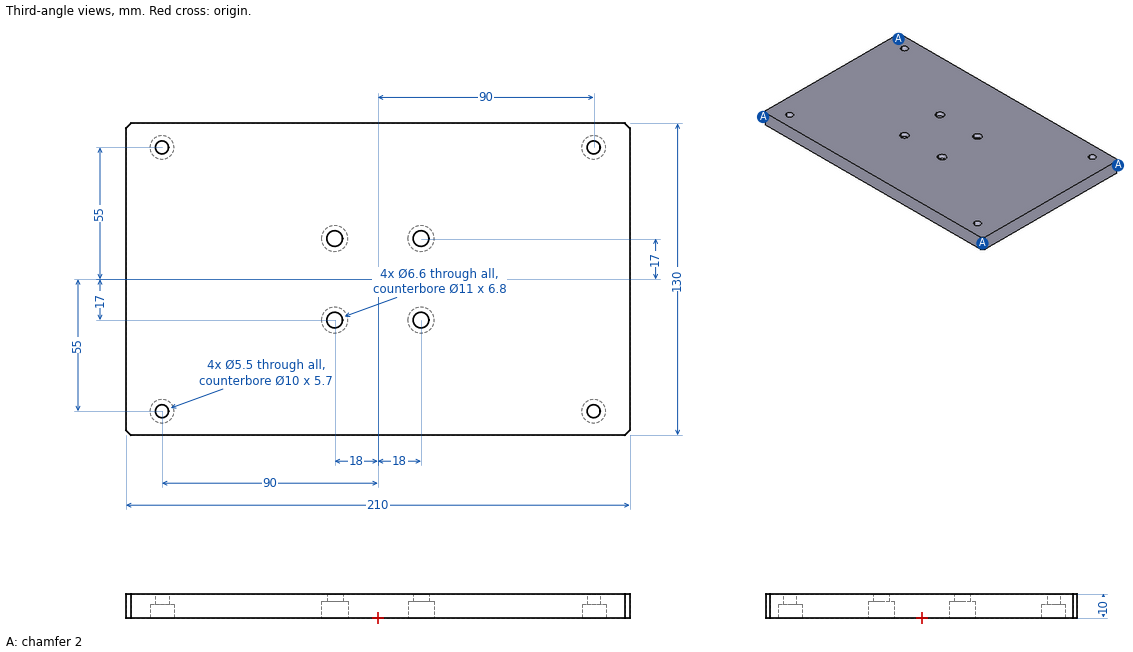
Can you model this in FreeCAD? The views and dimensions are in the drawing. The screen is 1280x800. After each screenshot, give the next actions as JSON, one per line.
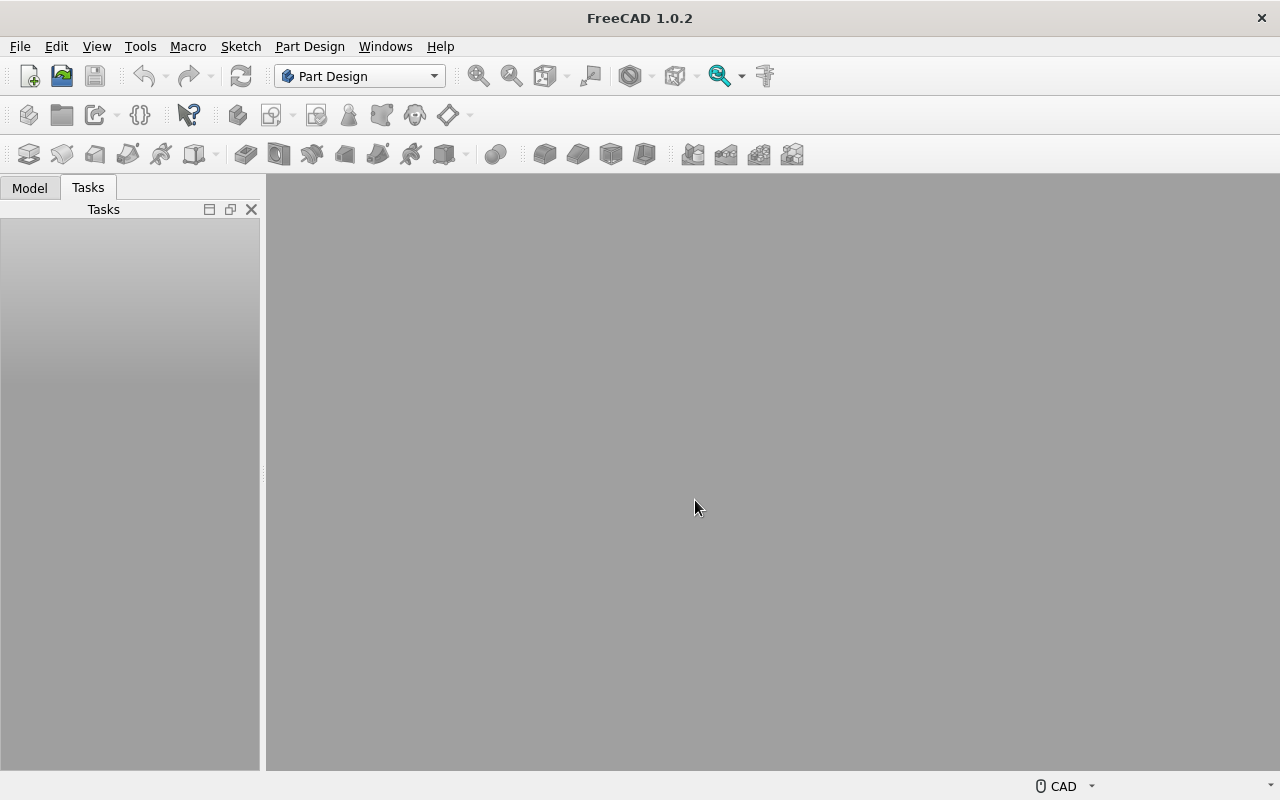
{"action": "left_click", "coordinate": [29, 76]}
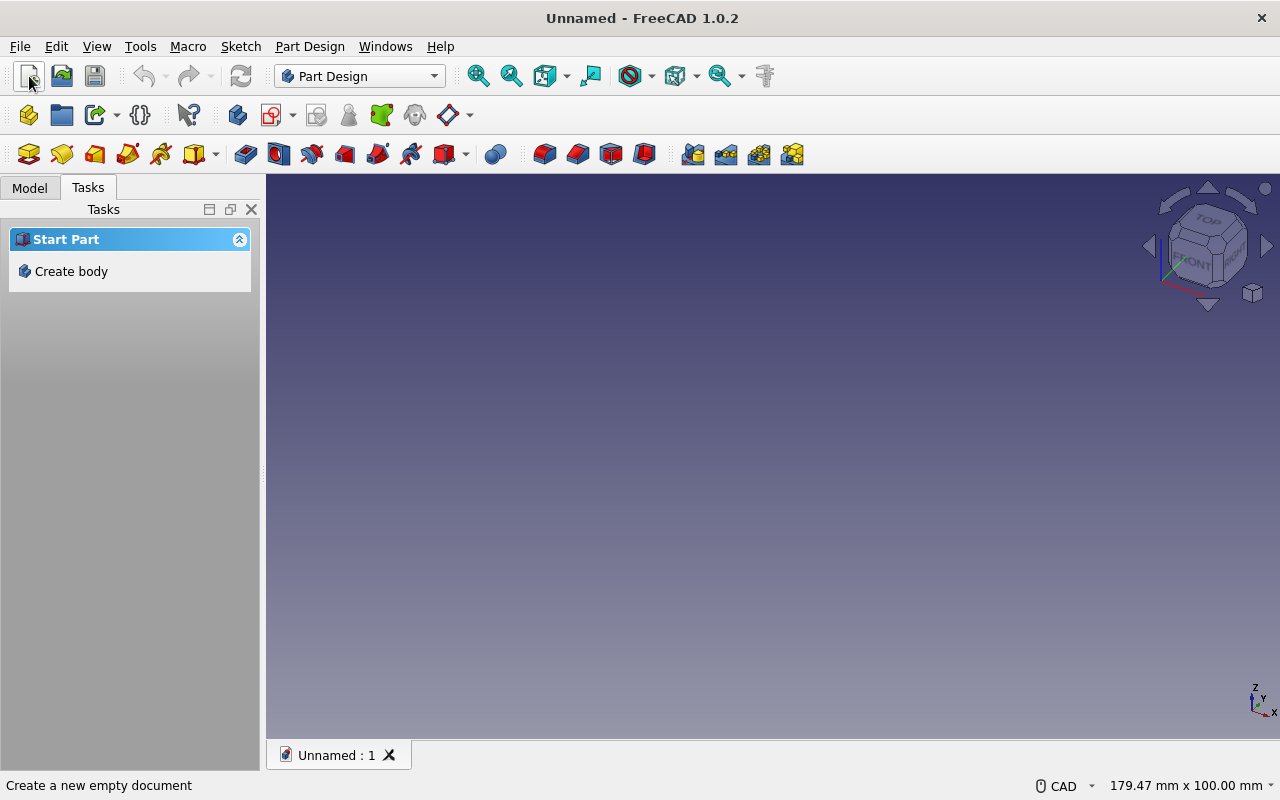
{"action": "left_click", "coordinate": [270, 116]}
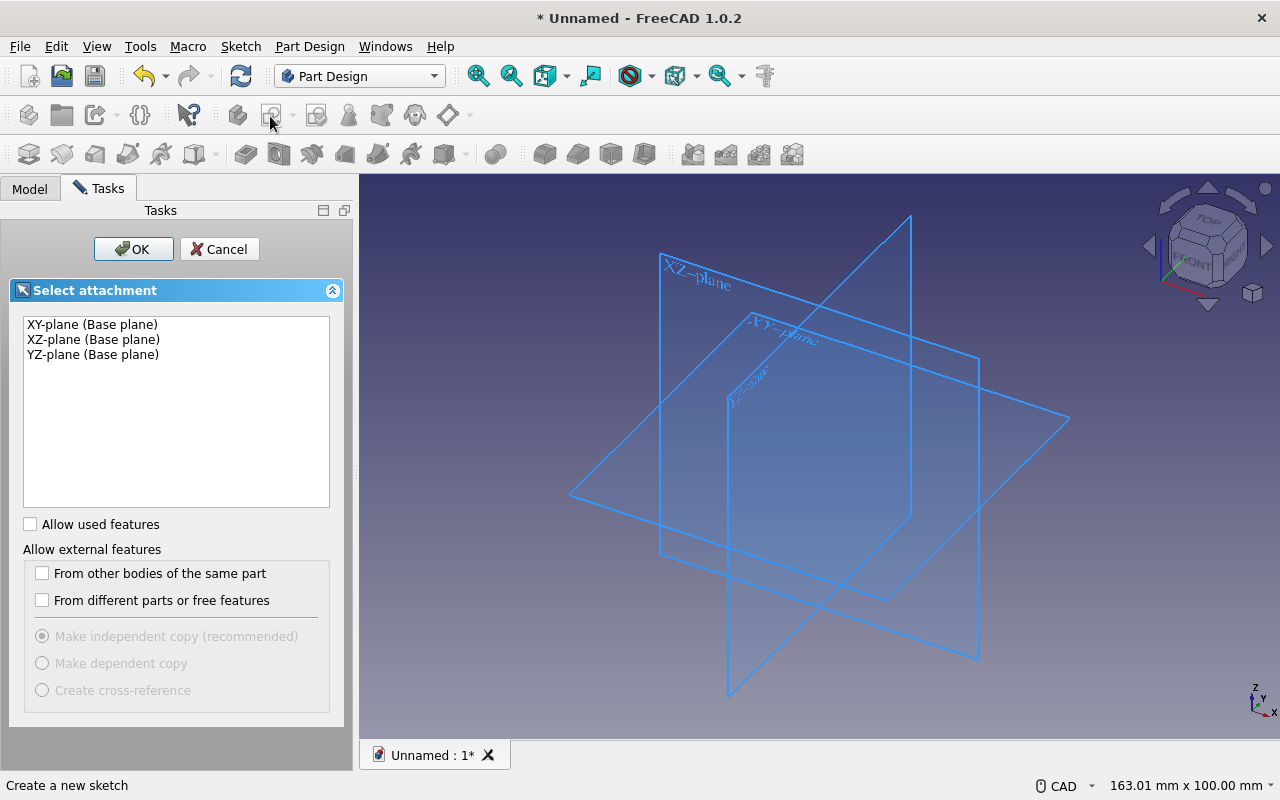
{"action": "left_click", "coordinate": [84, 324]}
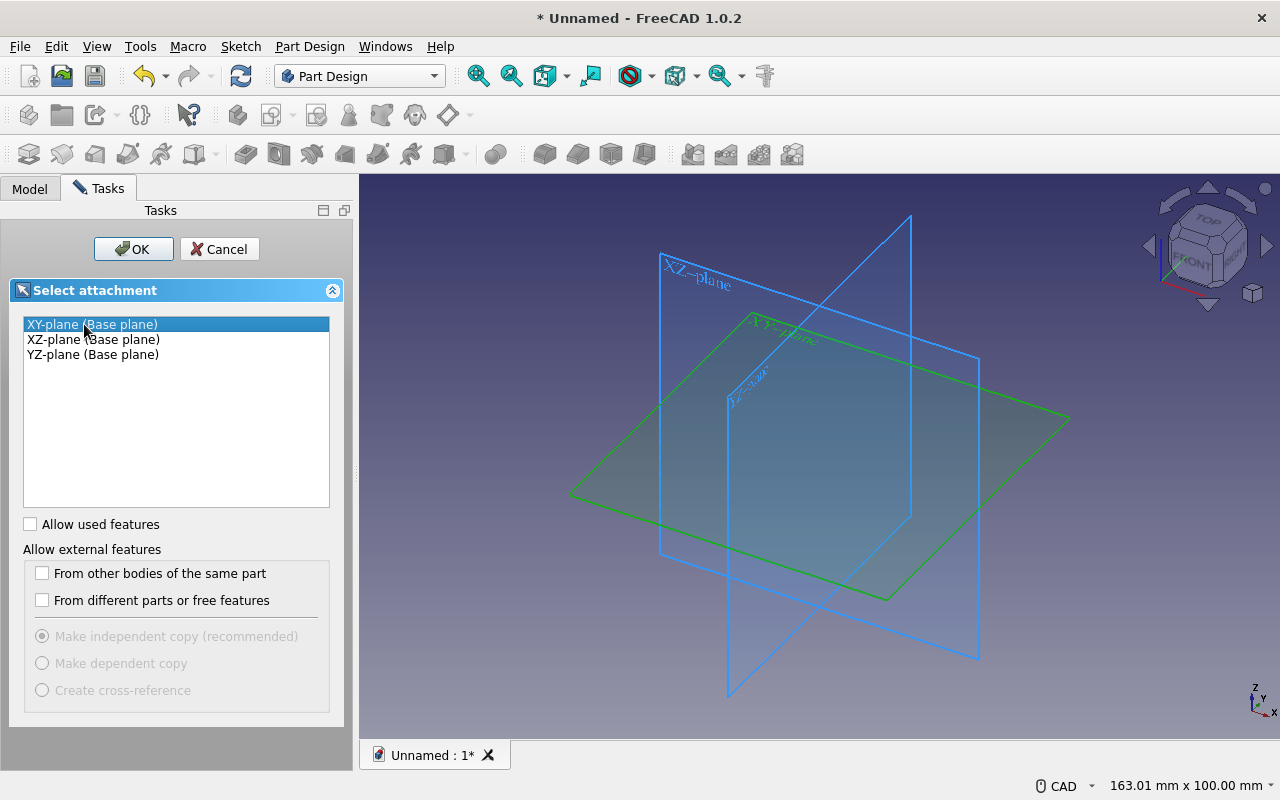
{"action": "left_click", "coordinate": [134, 249]}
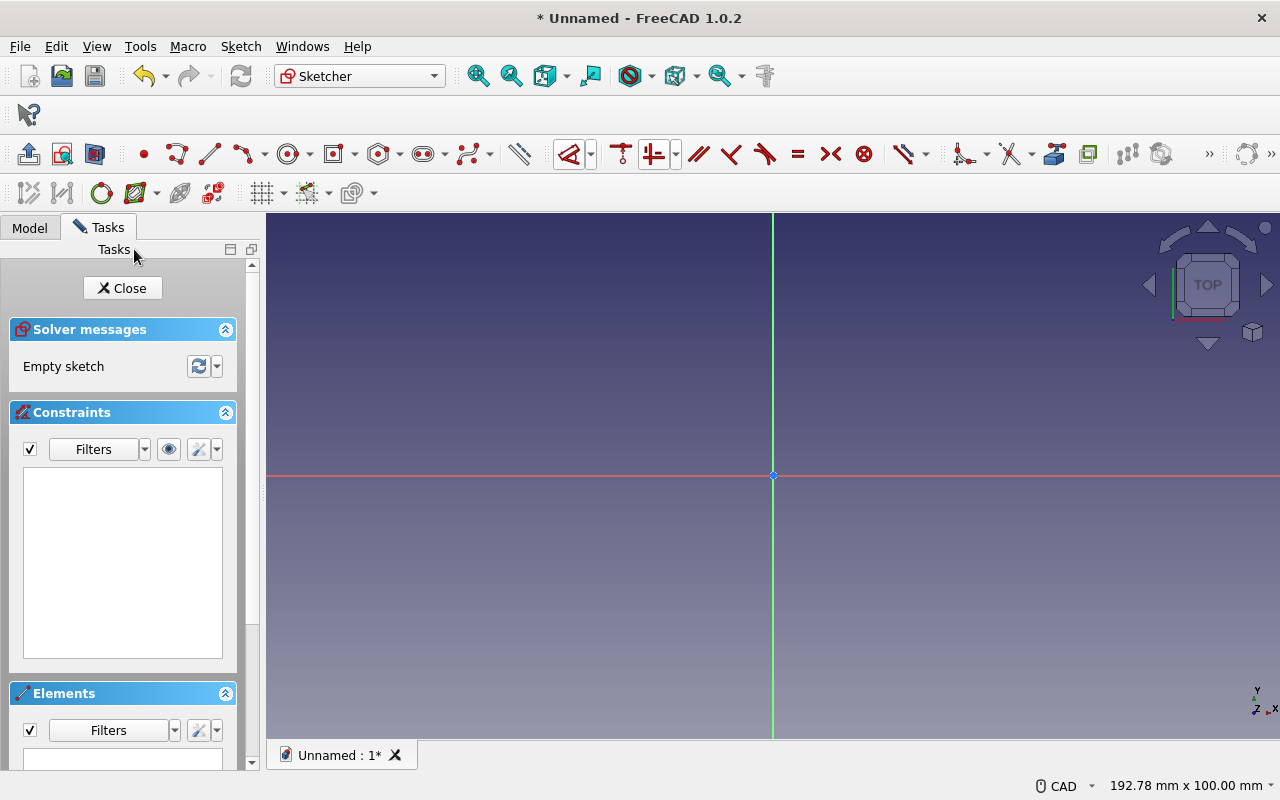
{"action": "scroll", "coordinate": [649, 476], "scroll_direction": "down", "scroll_amount": 4}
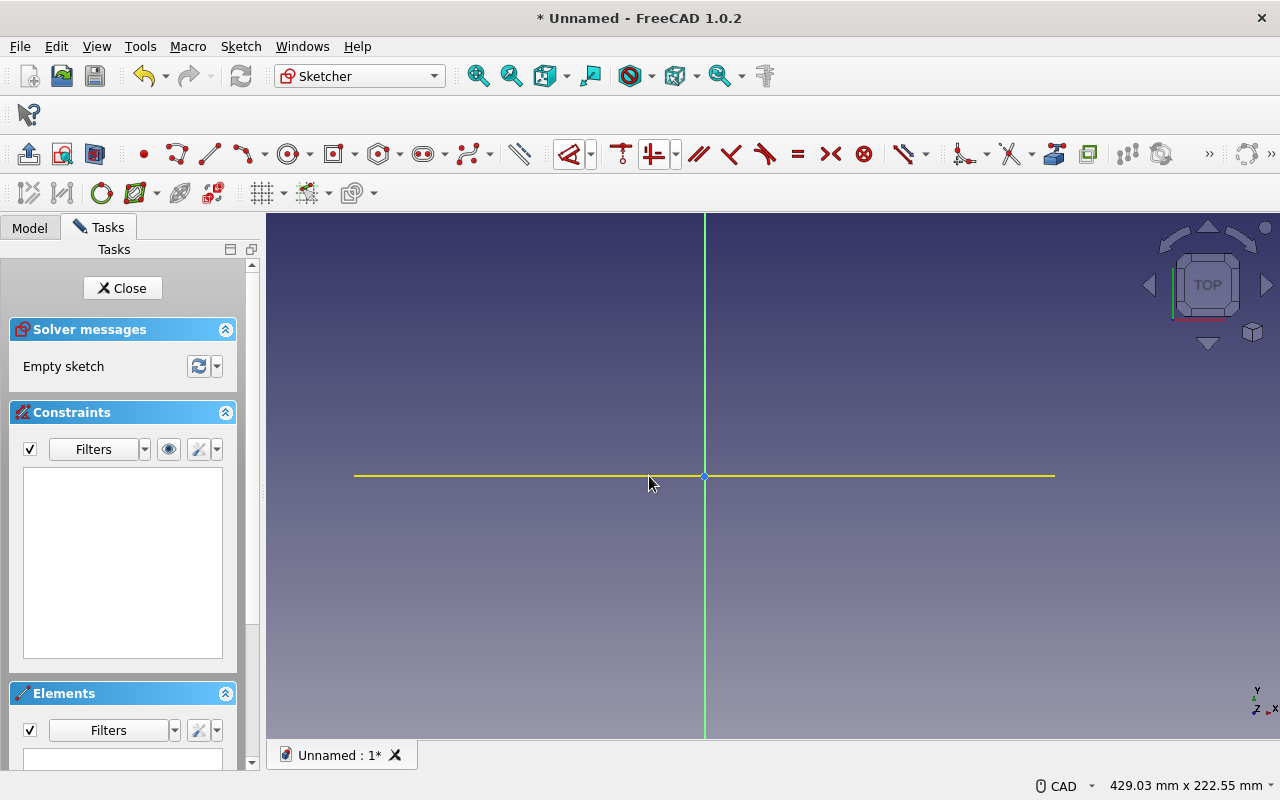
{"action": "key", "text": "g v"}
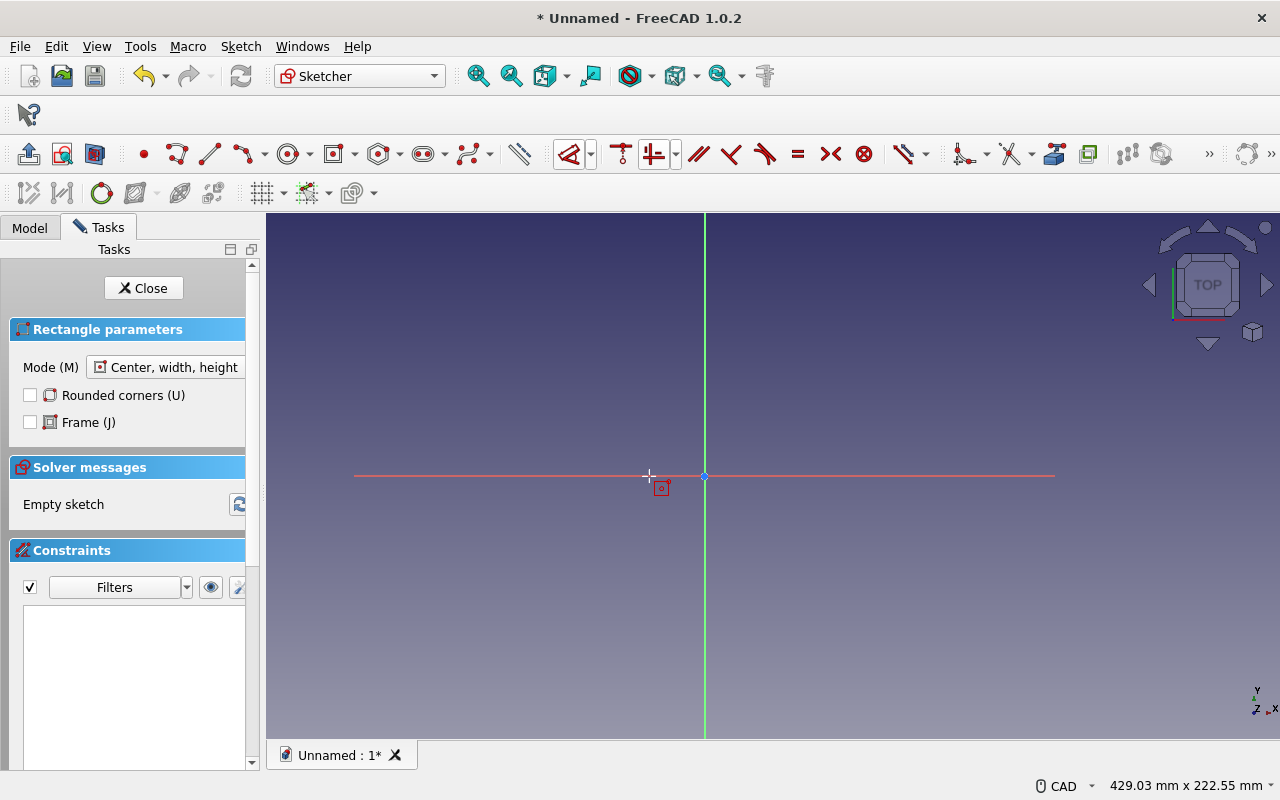
{"action": "left_click", "coordinate": [705, 476]}
{"action": "mouse_move", "coordinate": [953, 323]}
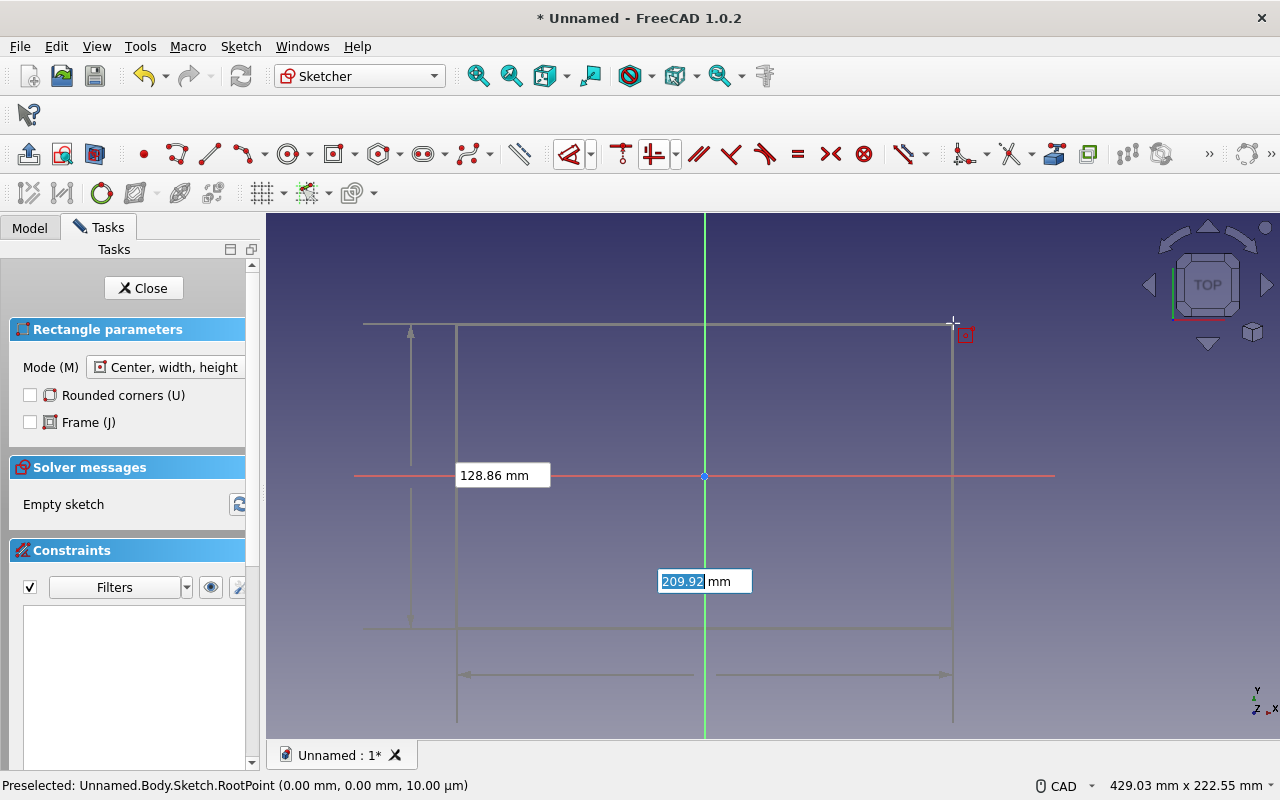
{"action": "type", "text": "210"}
{"action": "key", "text": "Tab"}
{"action": "type", "text": "130"}
{"action": "key", "text": "Return"}
{"action": "key", "text": "Escape"}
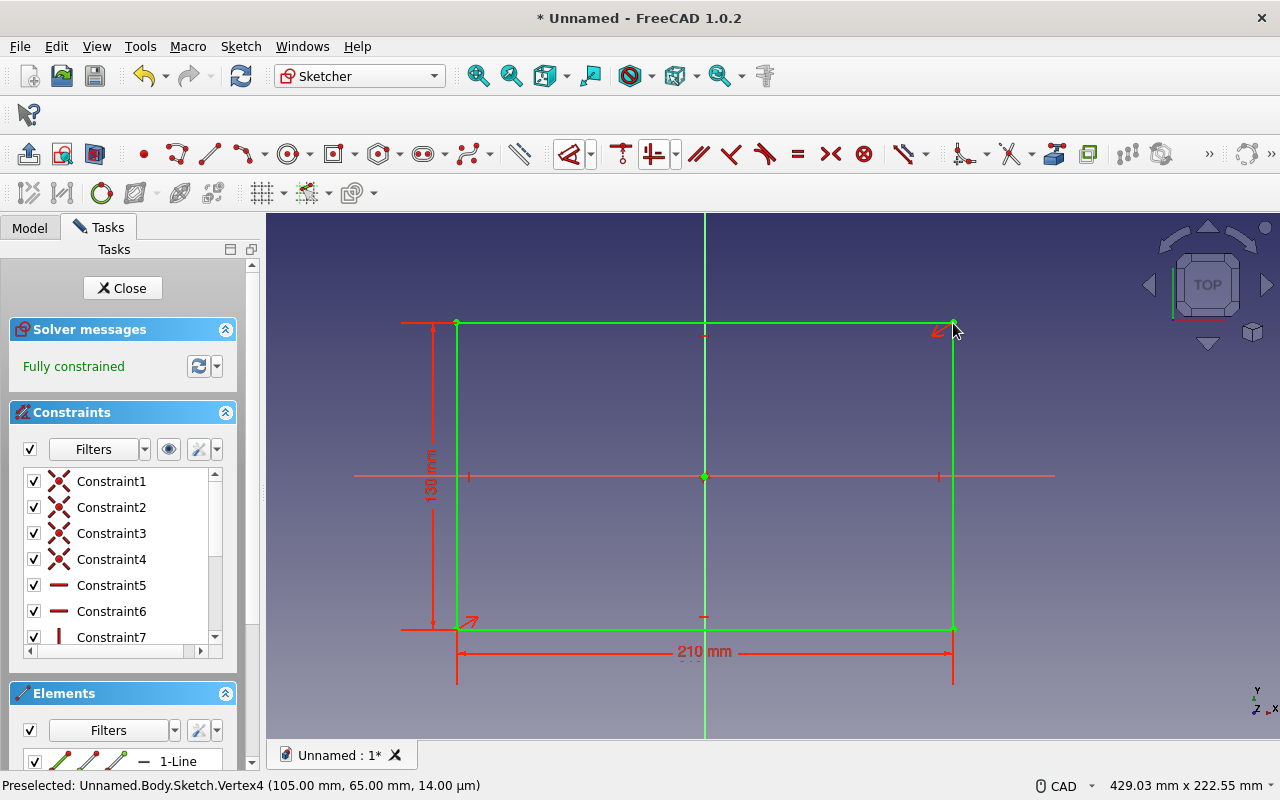
{"action": "left_click", "coordinate": [123, 288]}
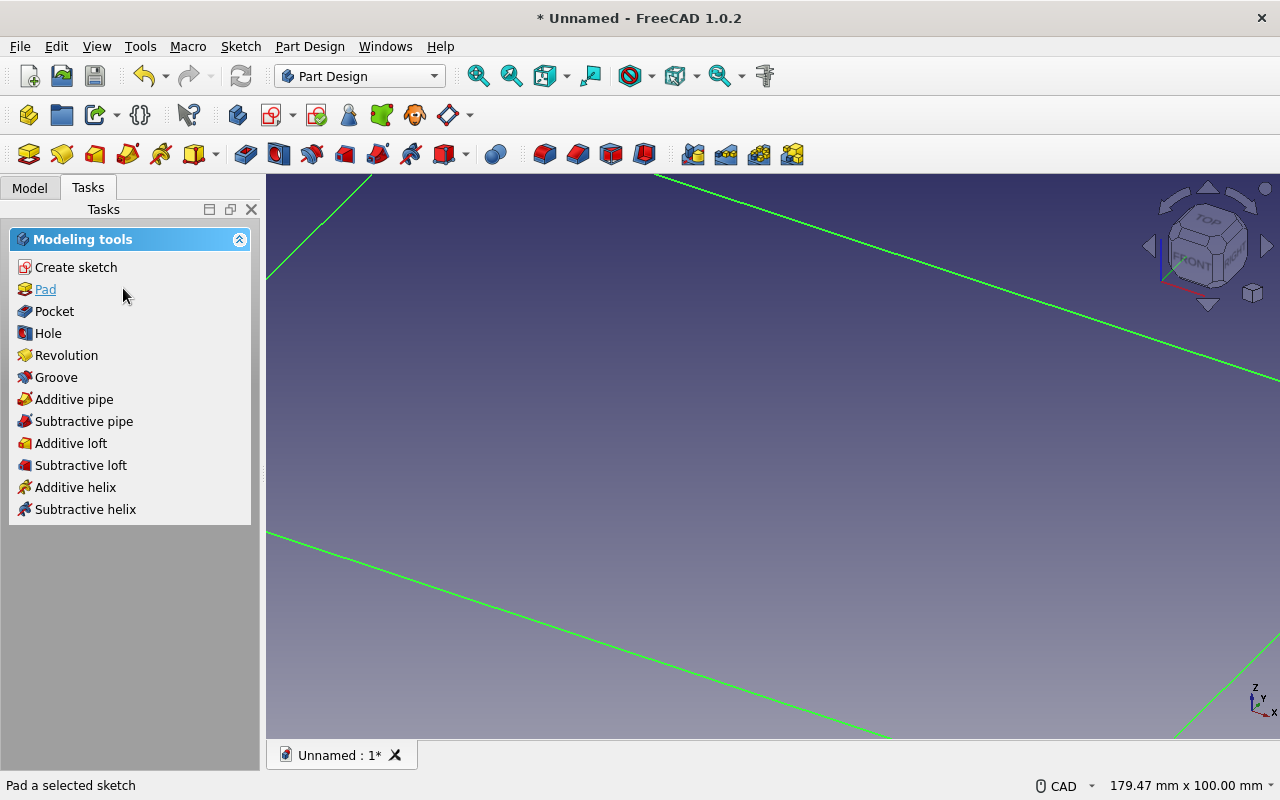
{"action": "left_click", "coordinate": [29, 154]}